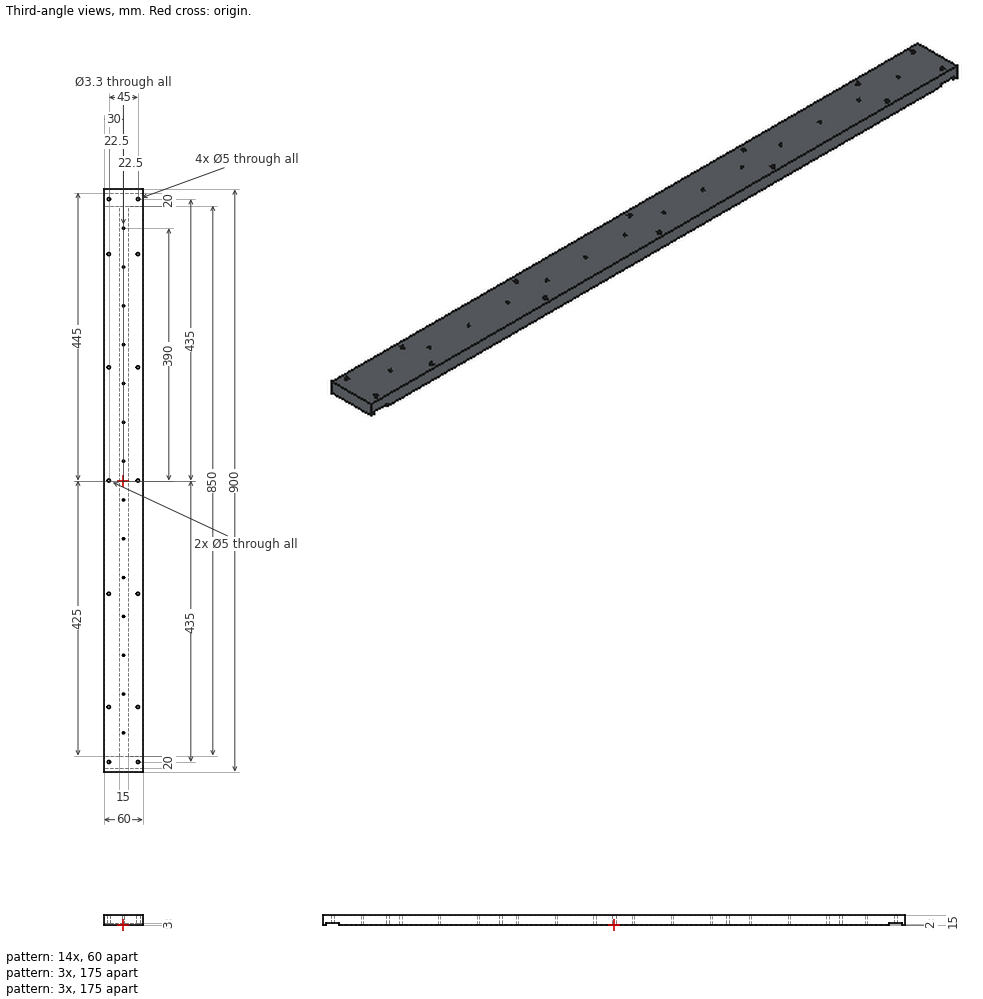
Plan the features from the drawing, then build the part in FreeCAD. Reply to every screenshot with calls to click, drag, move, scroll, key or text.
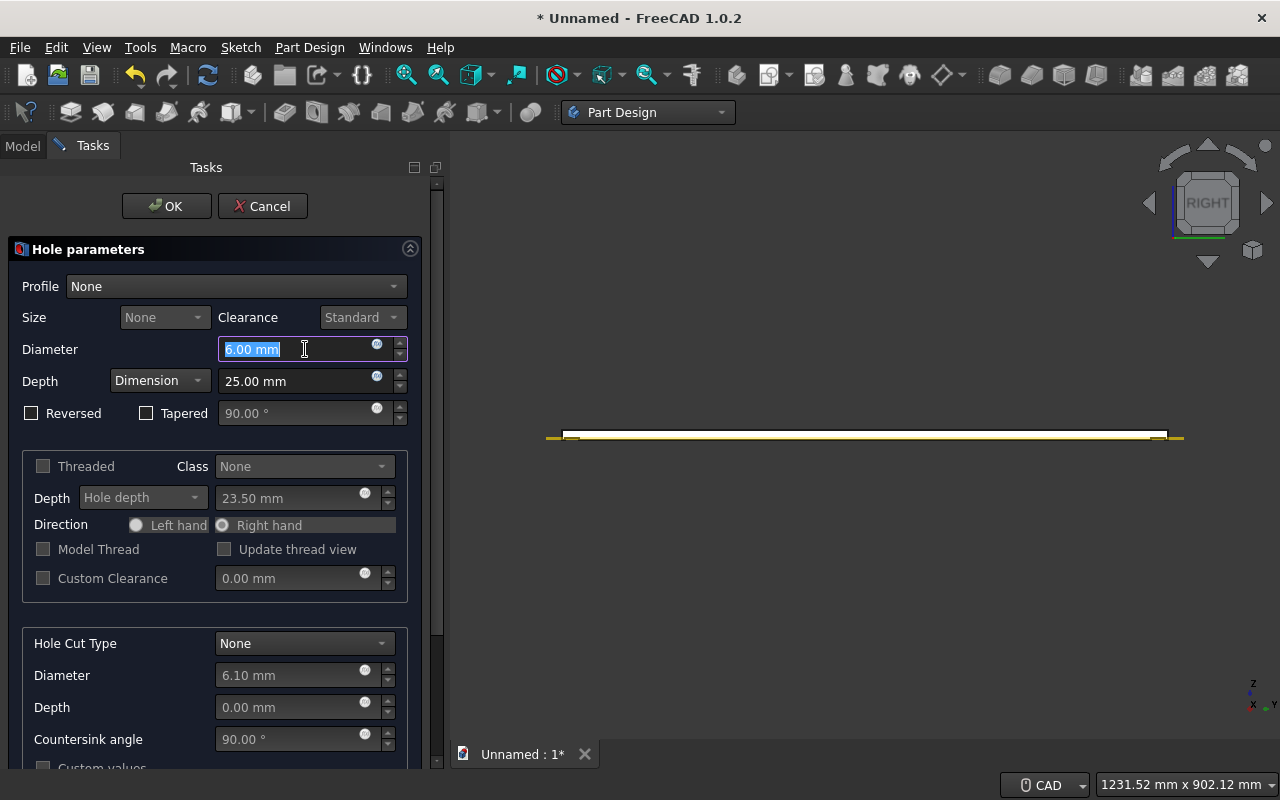
text(5)
key(Tab)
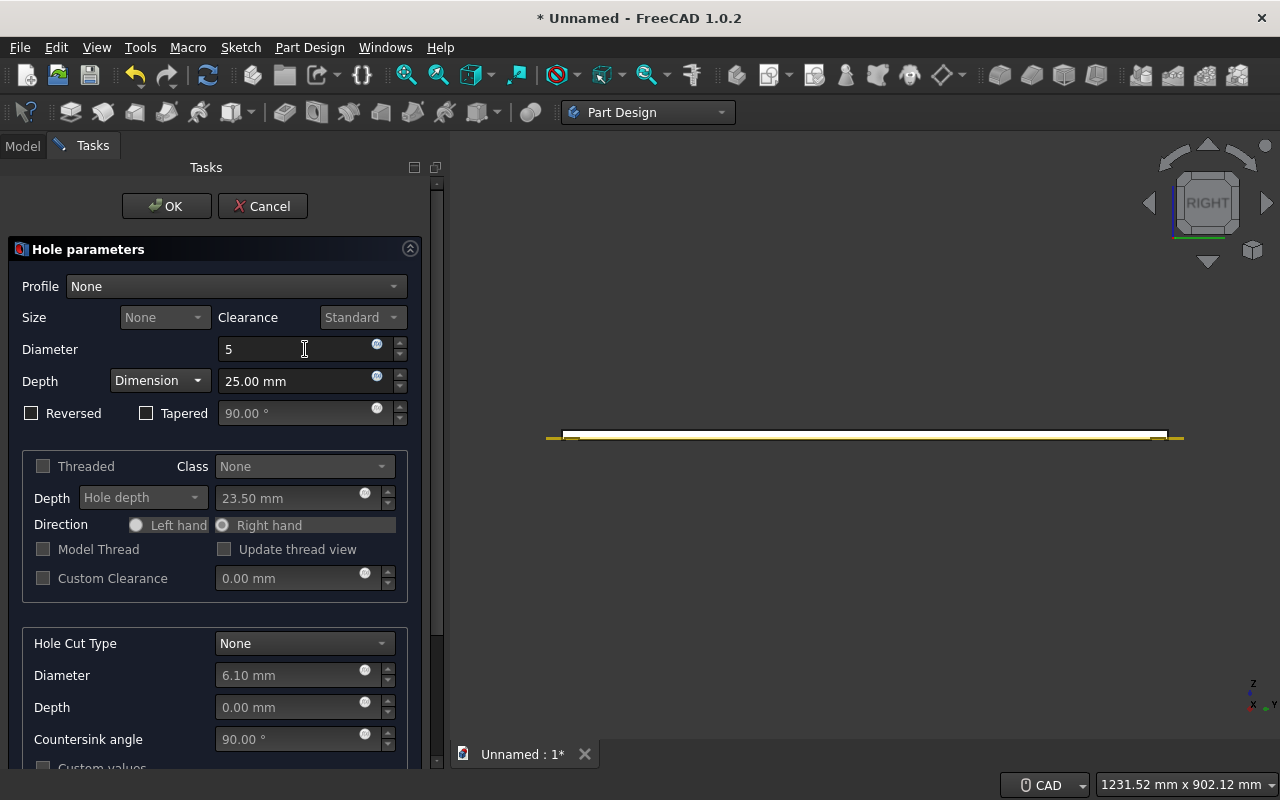
click(161, 380)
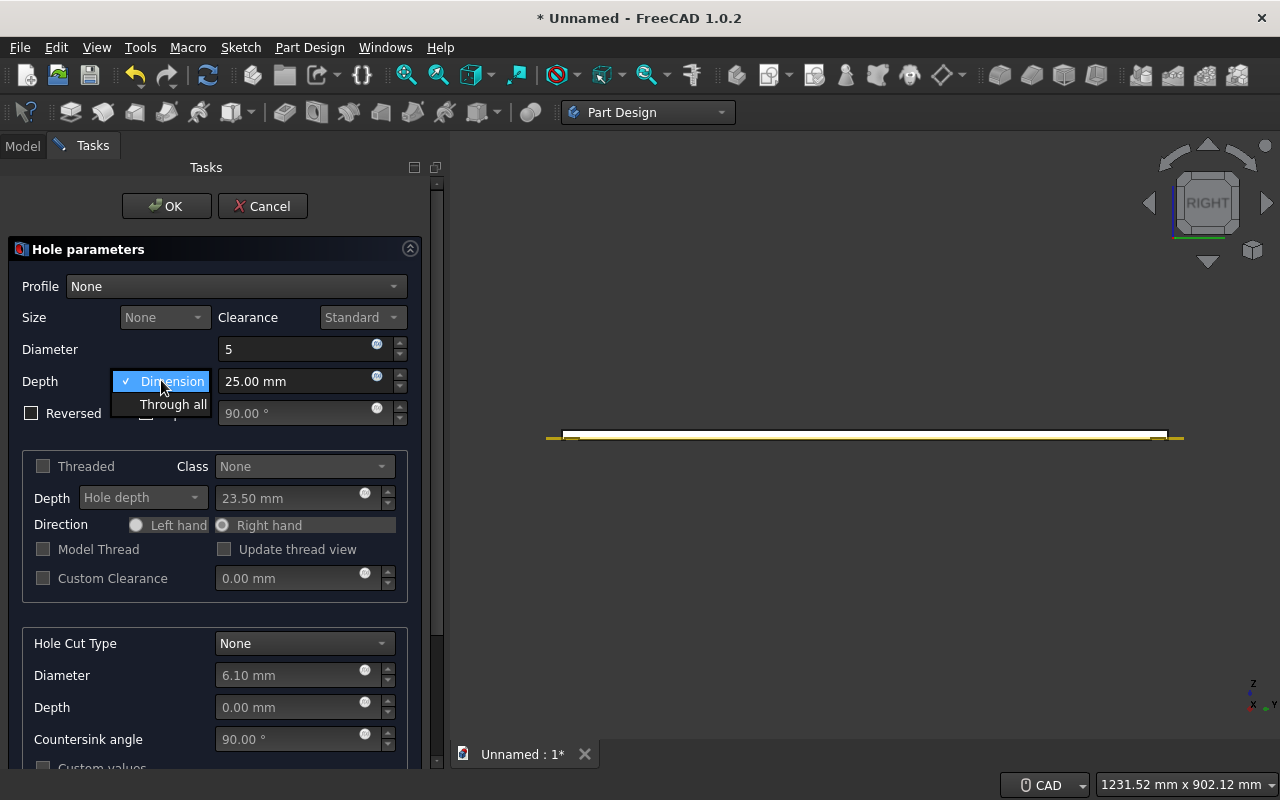
click(160, 404)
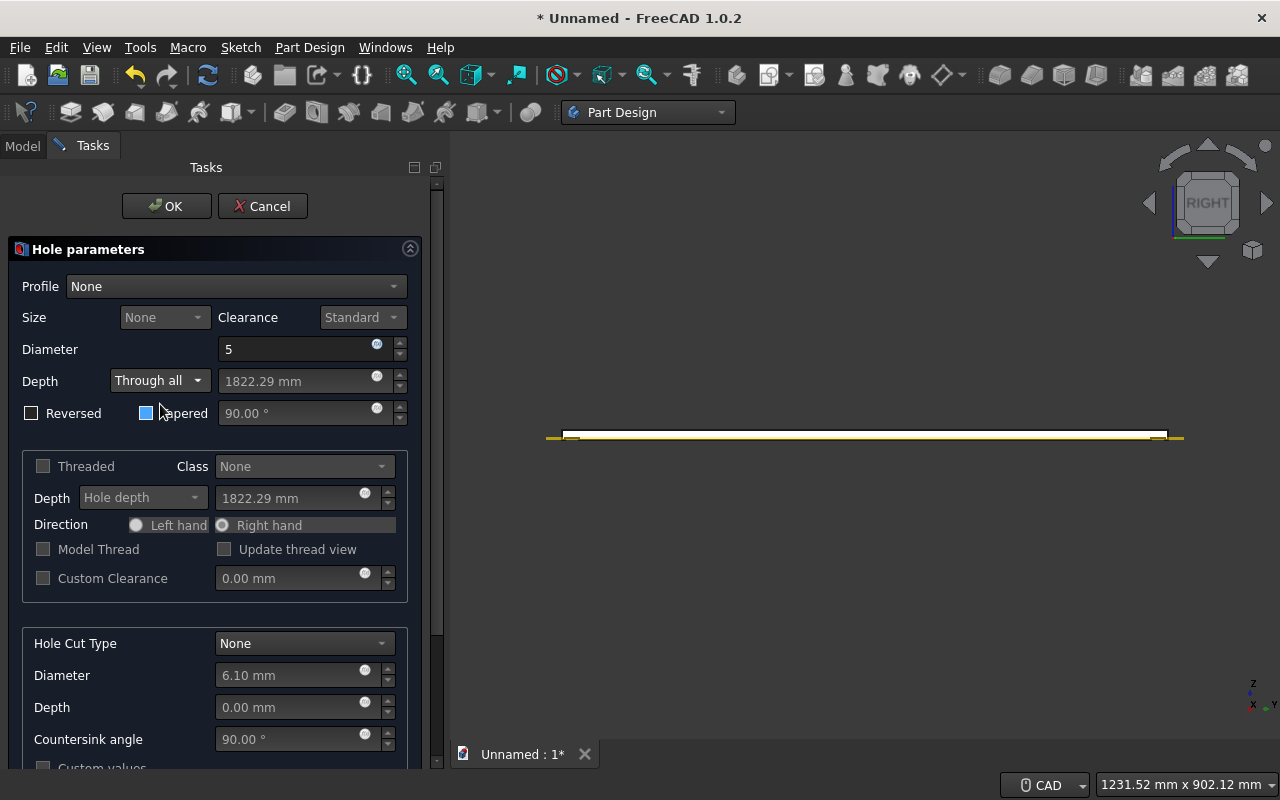
click(30, 413)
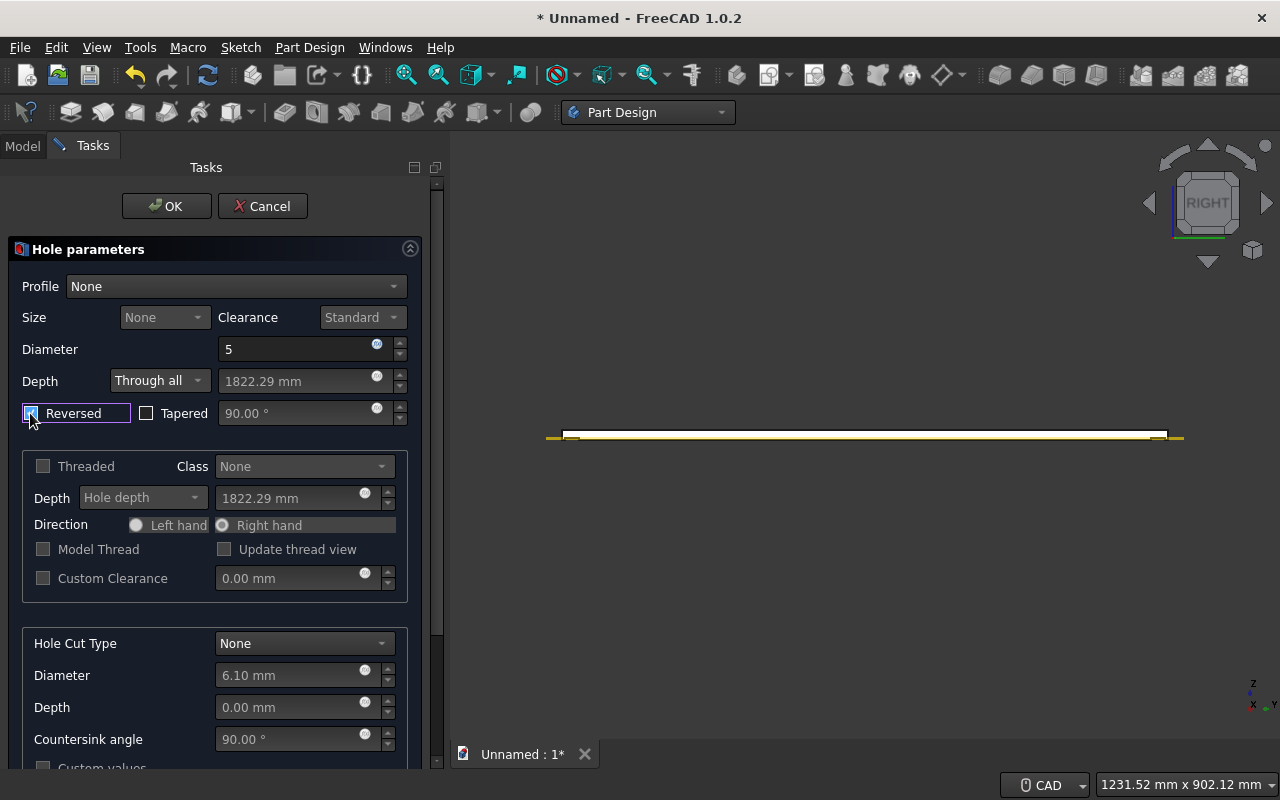
click(167, 206)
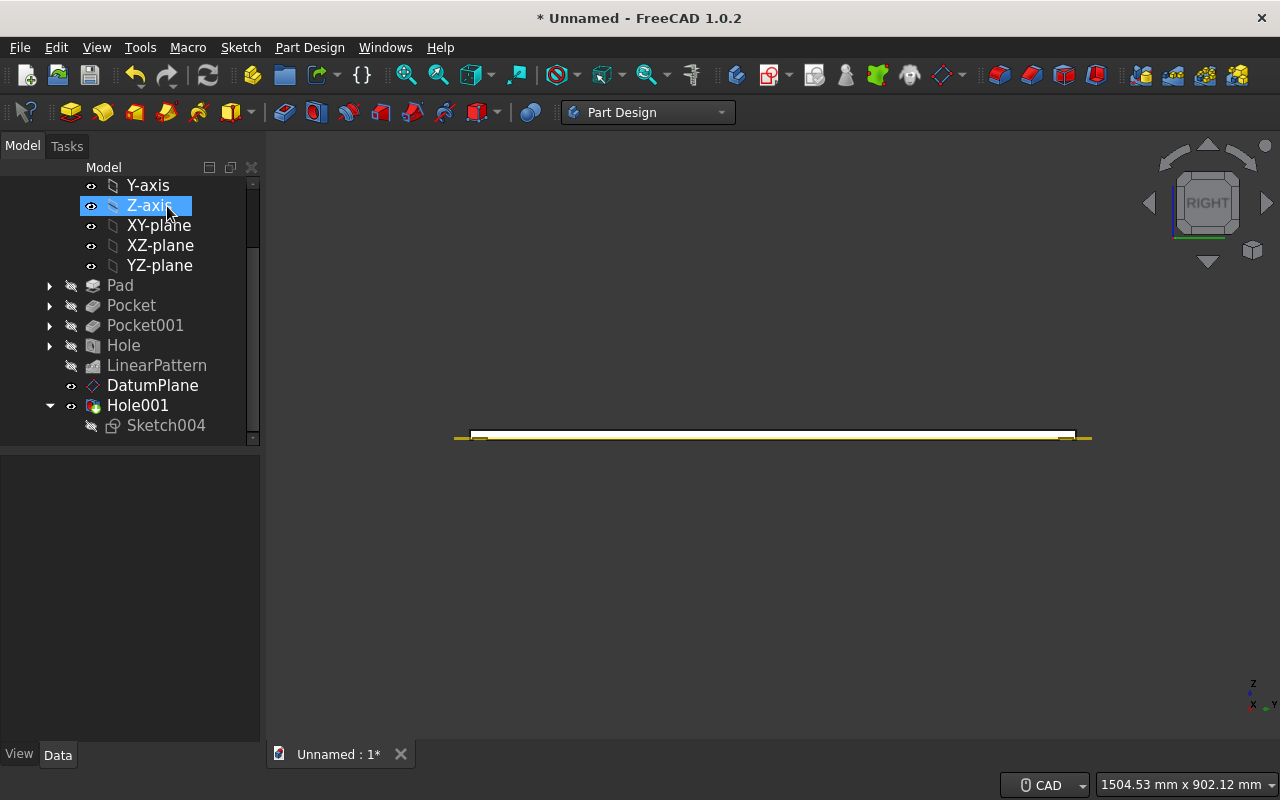
click(116, 386)
key(space)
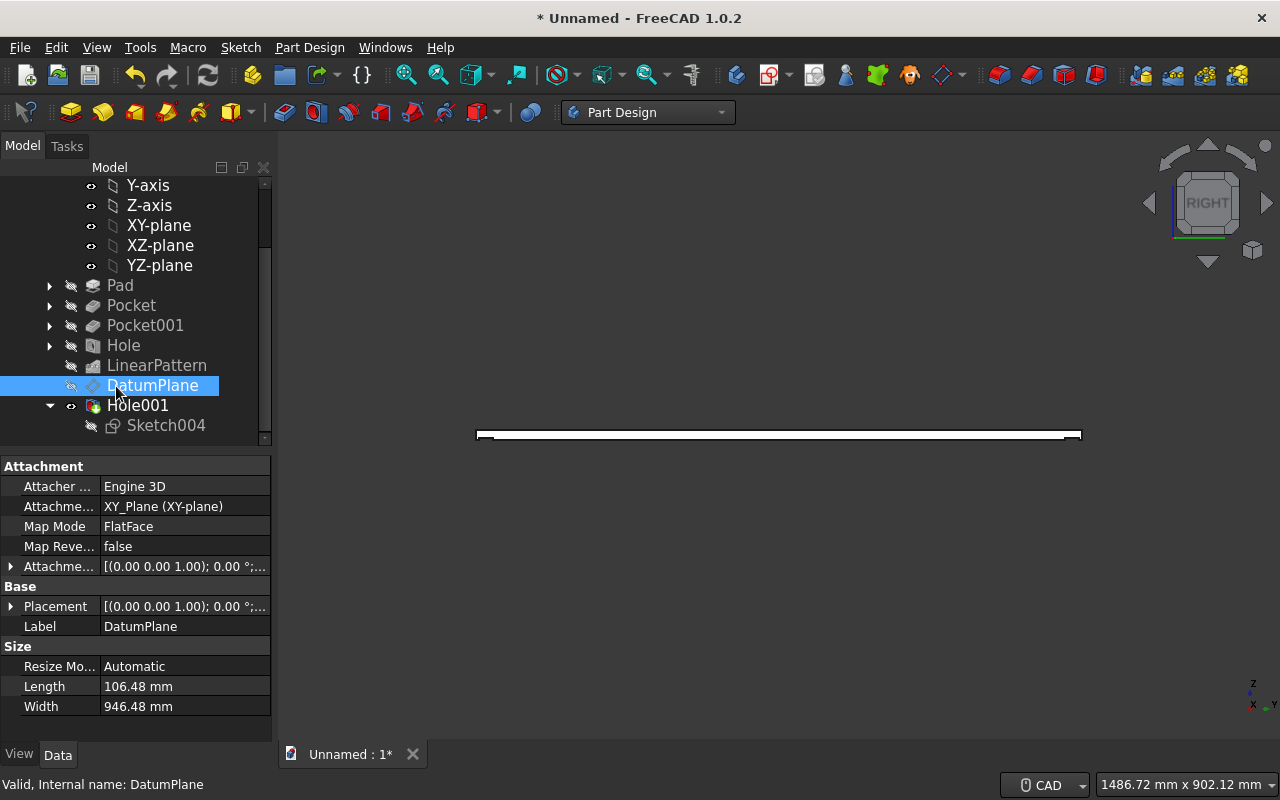
key(0)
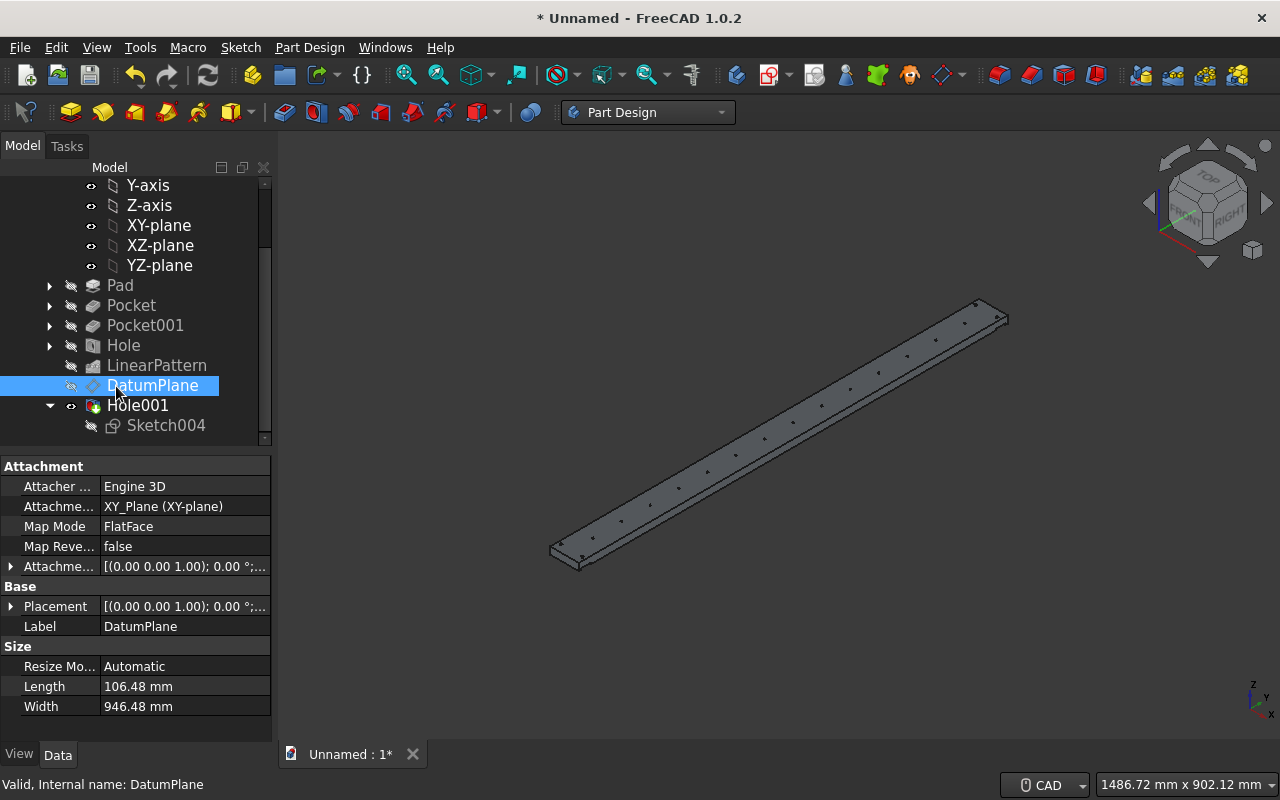
click(779, 430)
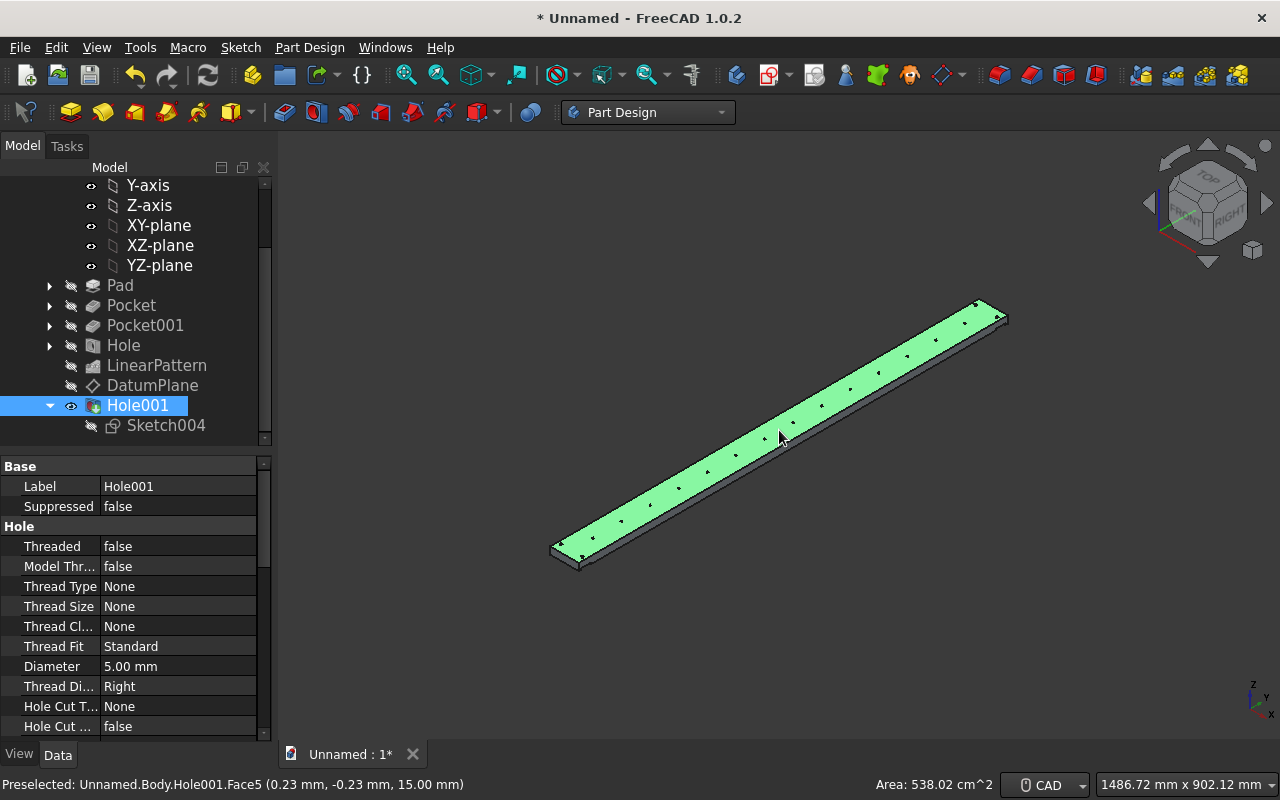
click(770, 76)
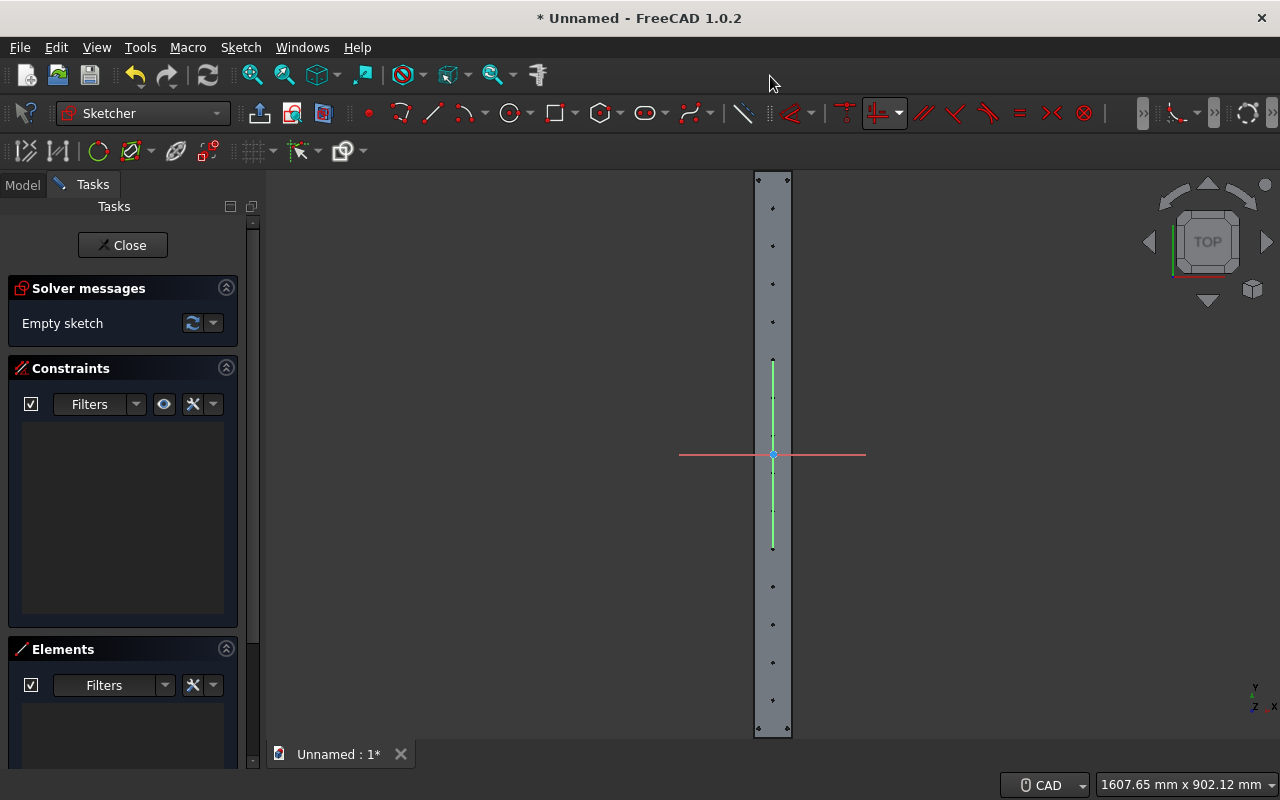
scroll(777, 454, up, 15)